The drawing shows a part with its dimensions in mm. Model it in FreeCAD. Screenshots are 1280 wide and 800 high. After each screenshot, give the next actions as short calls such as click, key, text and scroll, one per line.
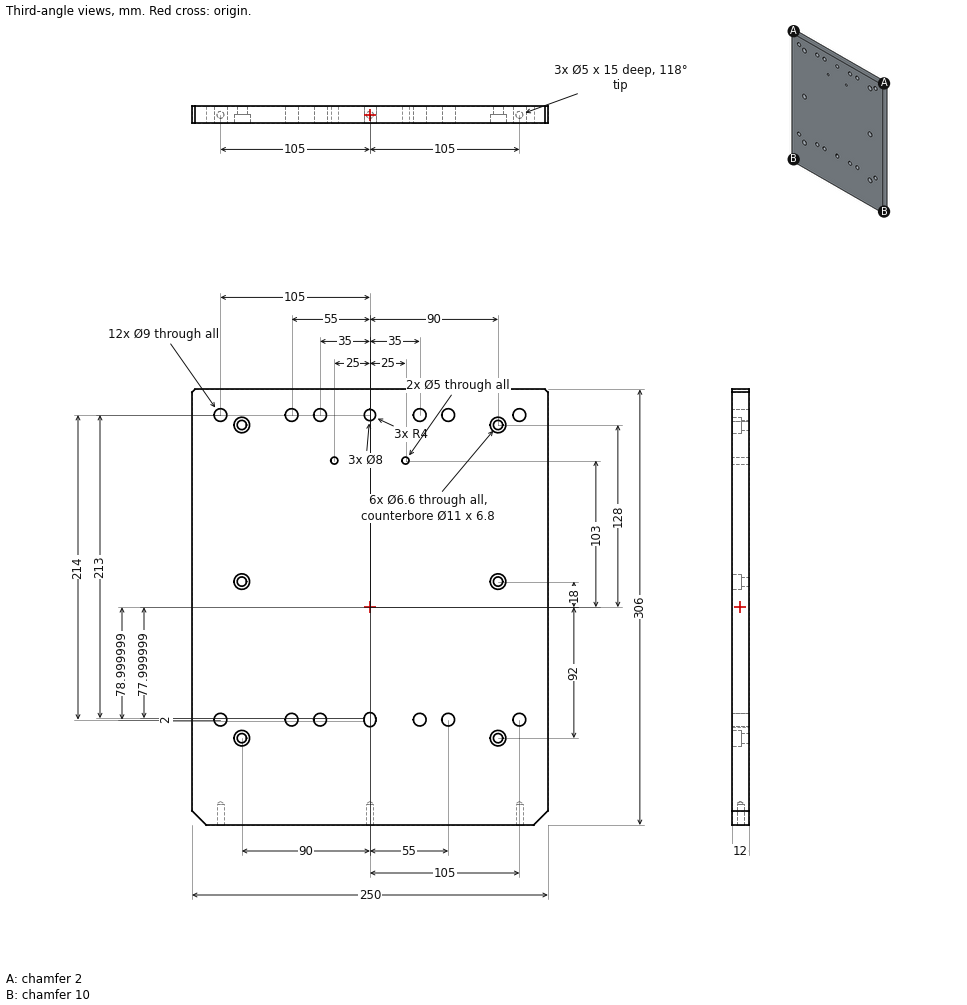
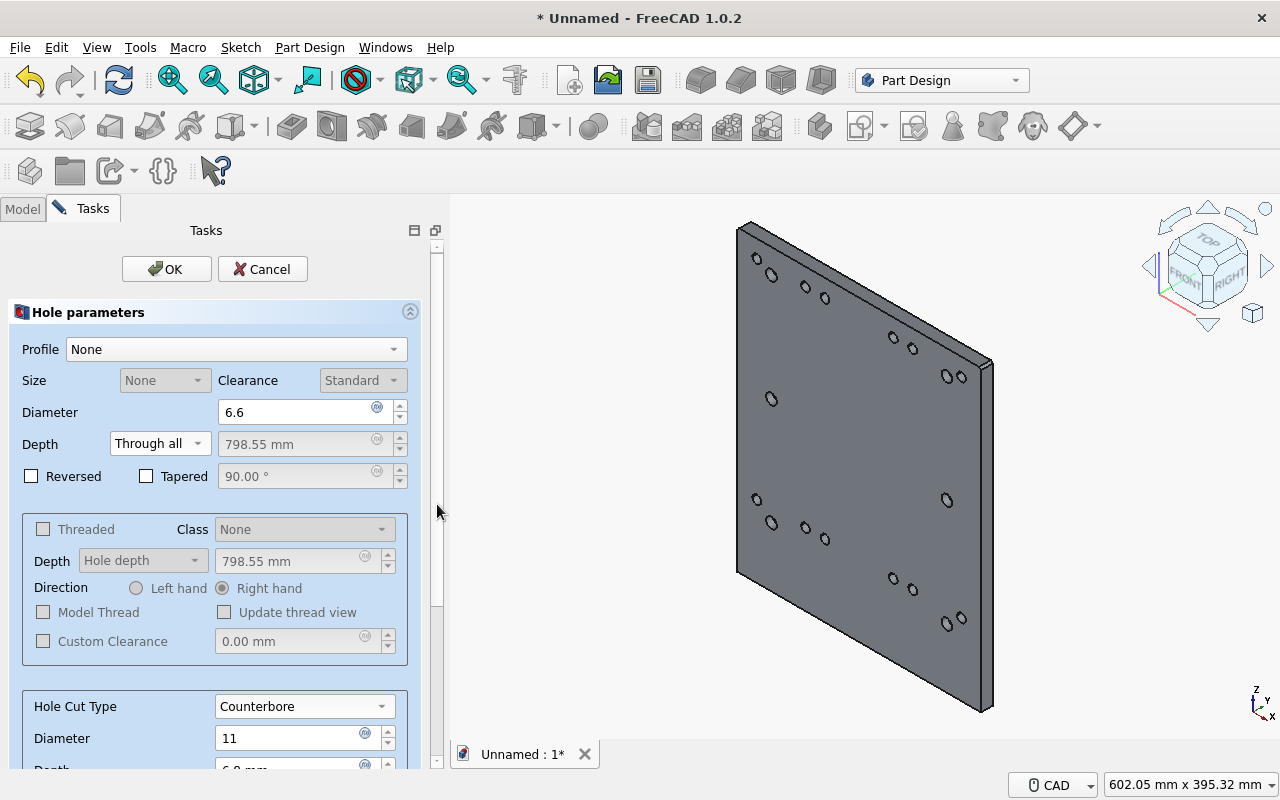
click(167, 269)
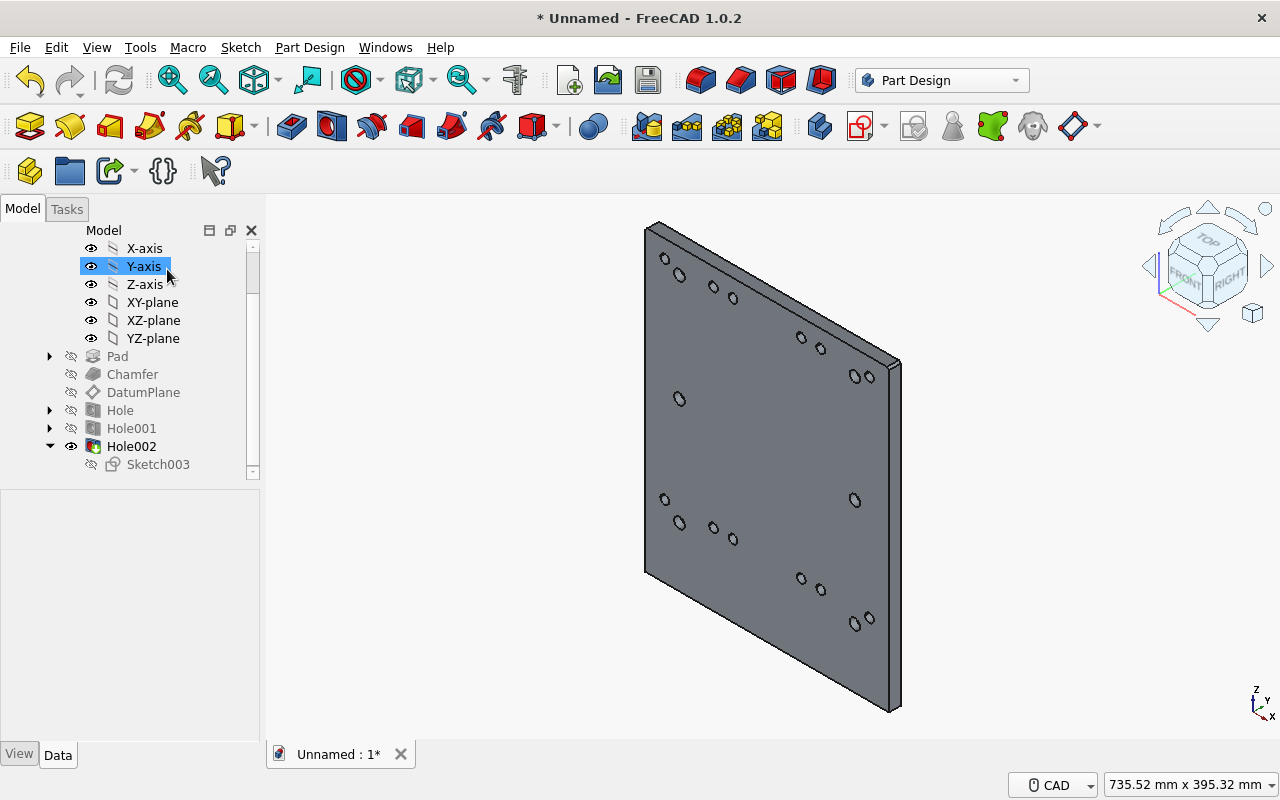
key(4)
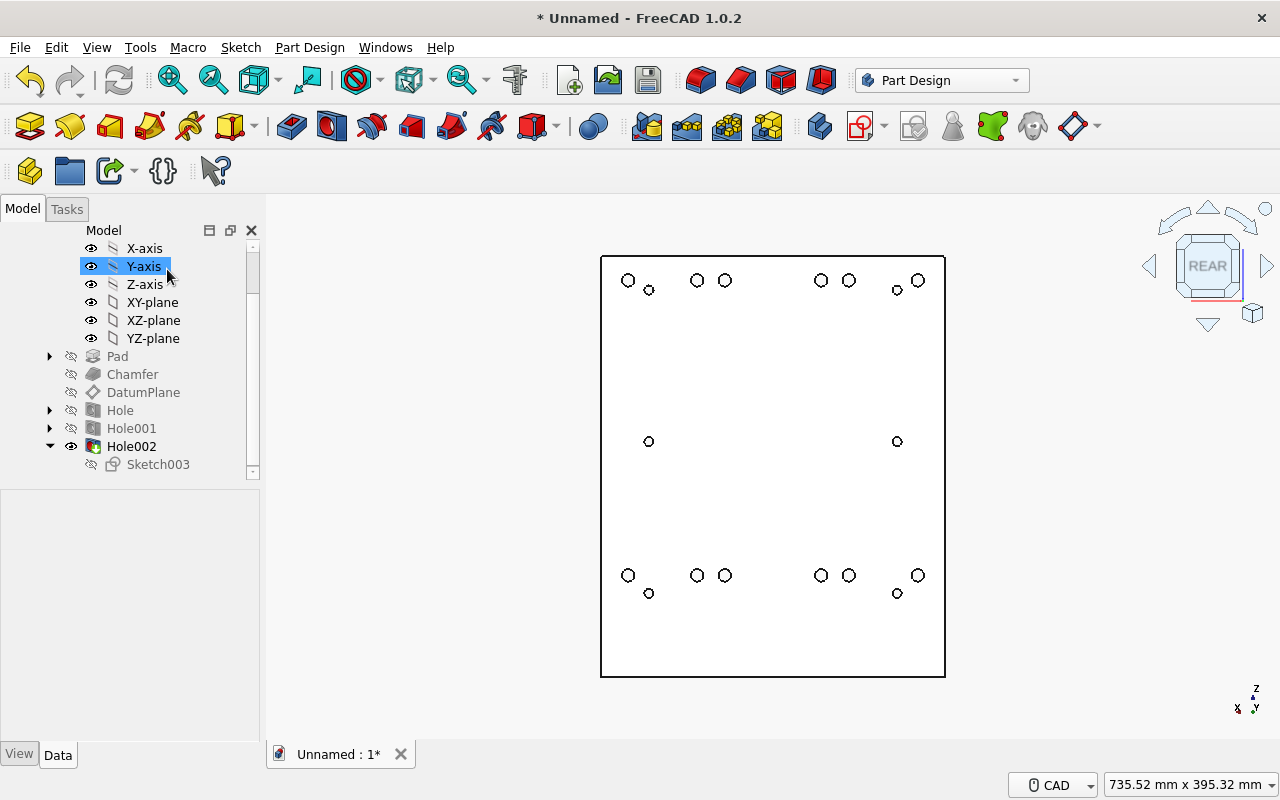
click(773, 405)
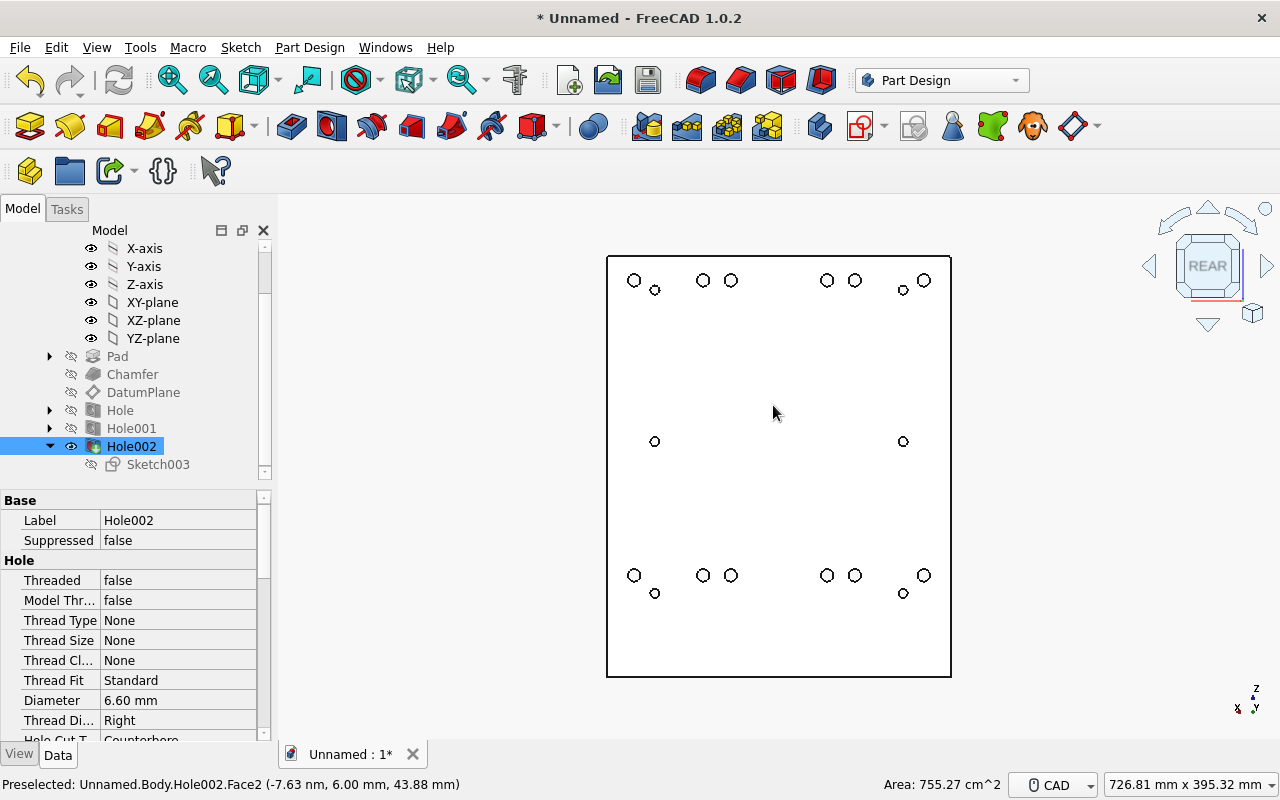
click(860, 126)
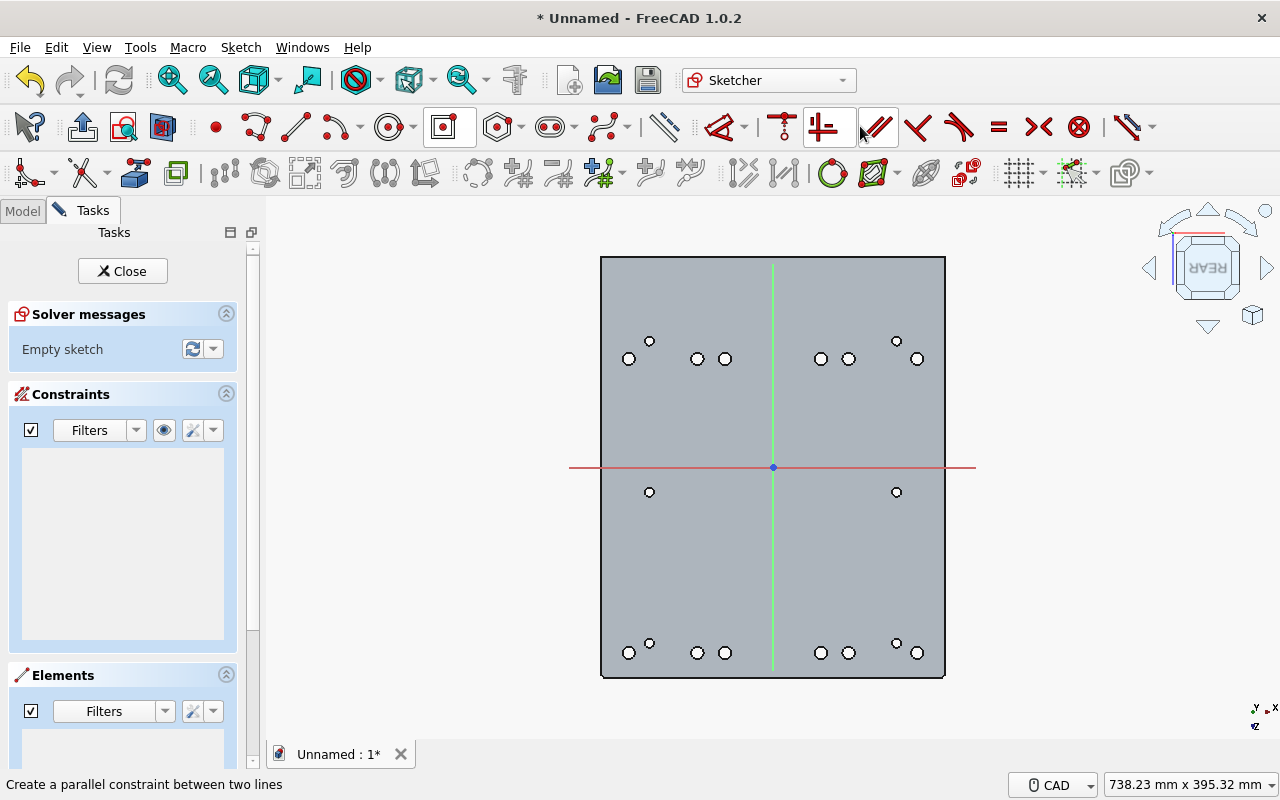
click(550, 128)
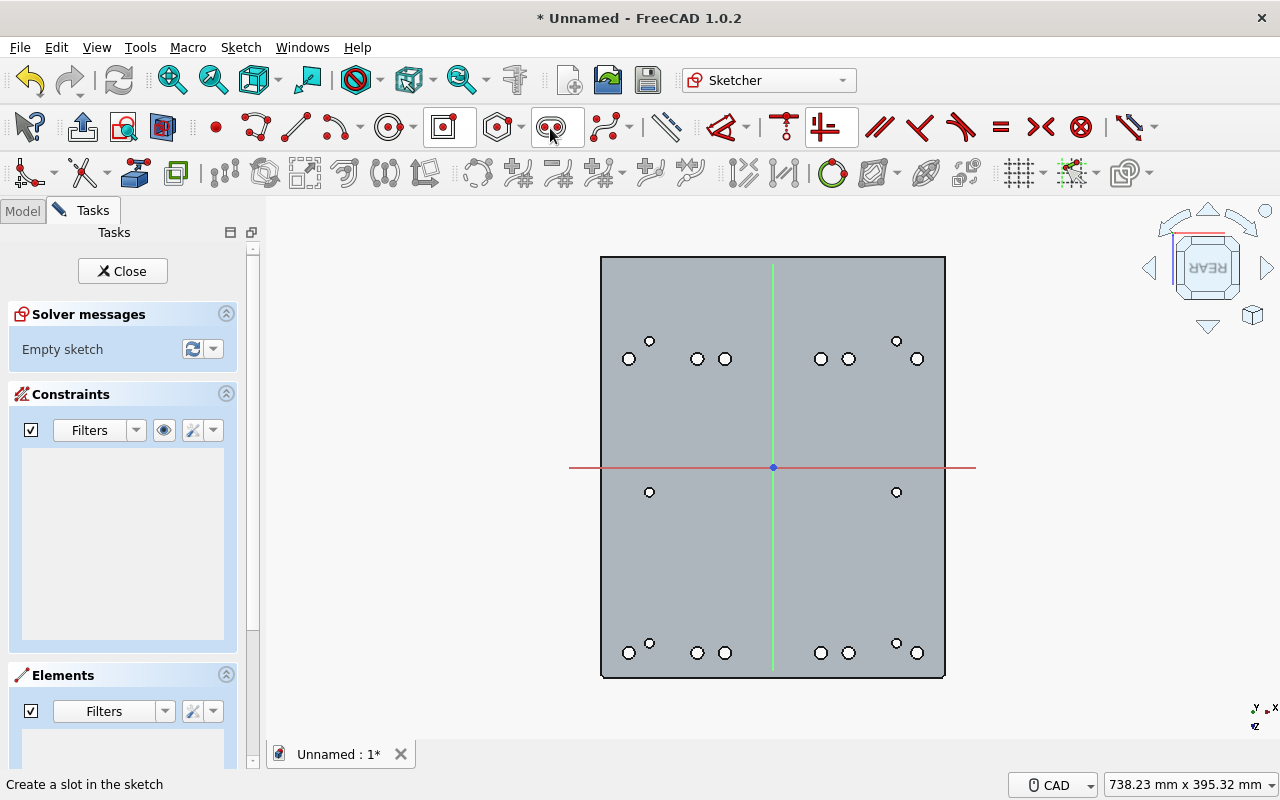
scroll(773, 360, up, 8)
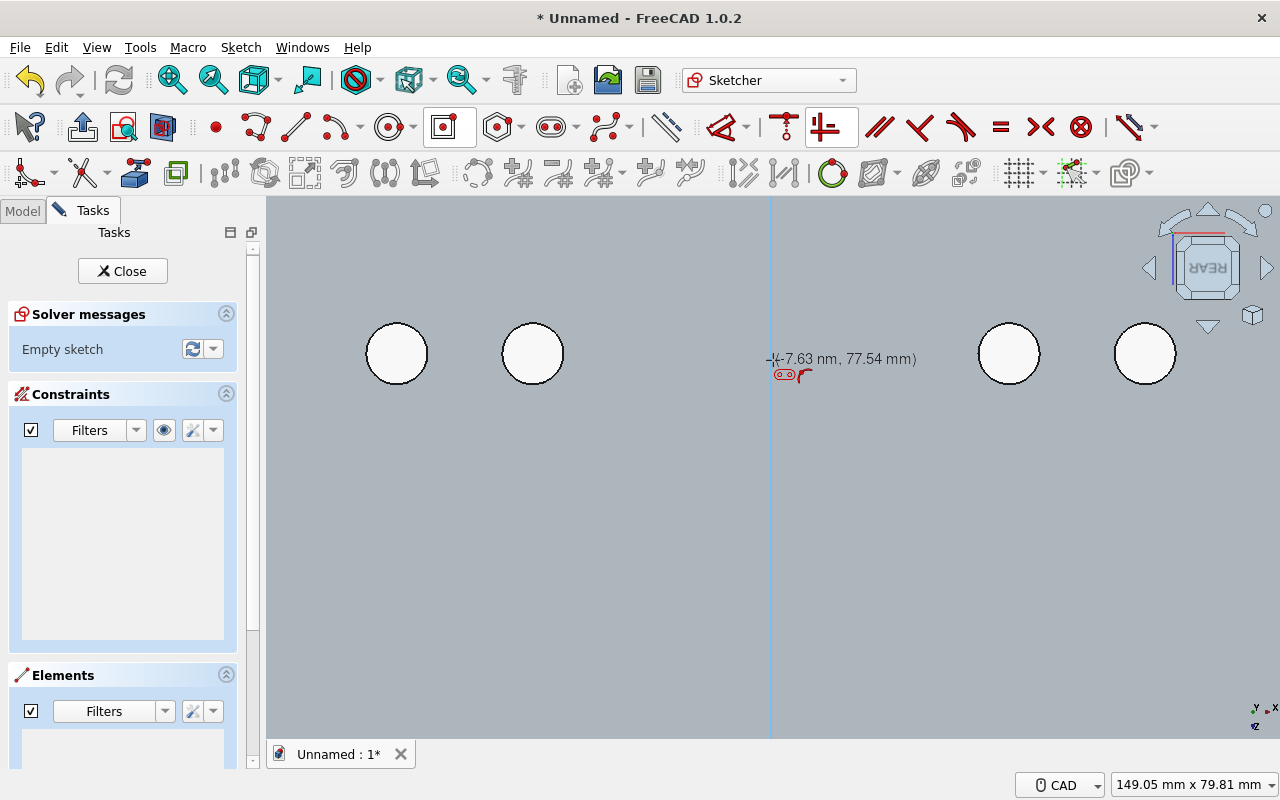
scroll(683, 268, down, 7)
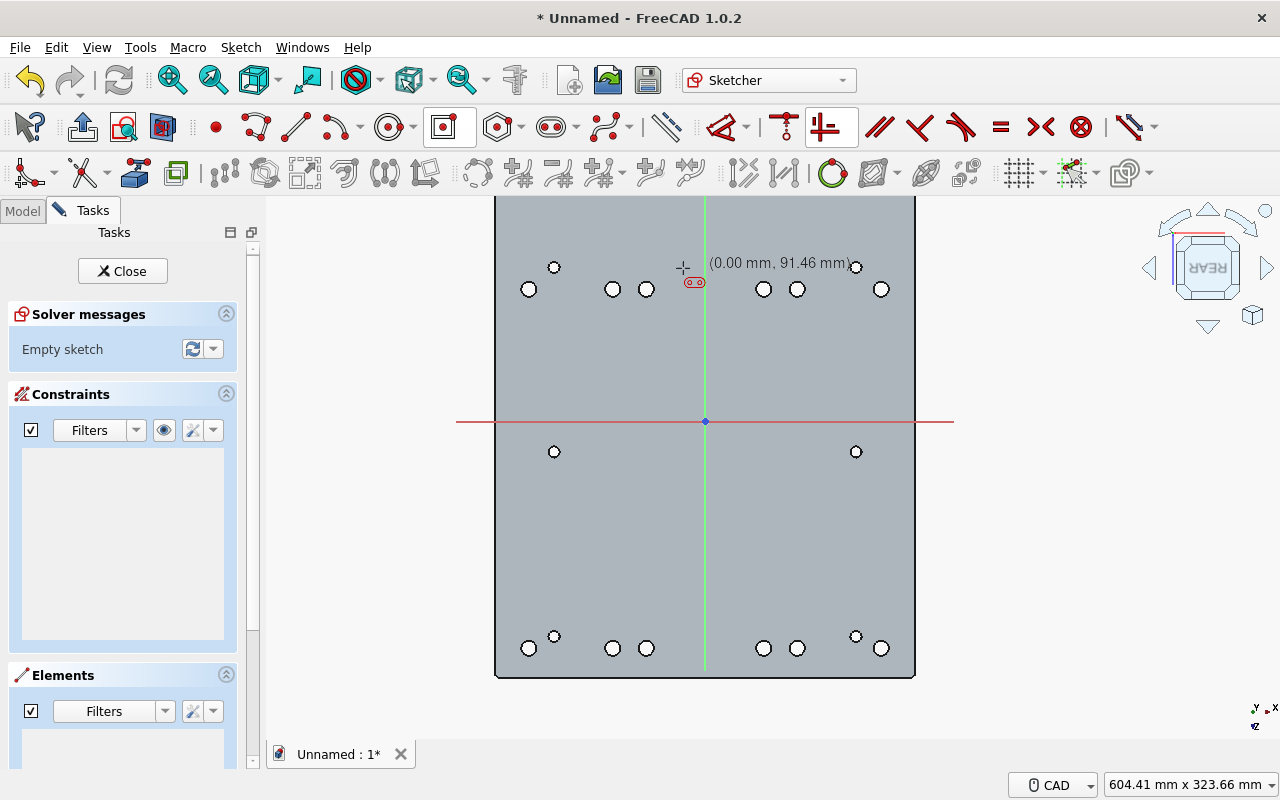
click(705, 291)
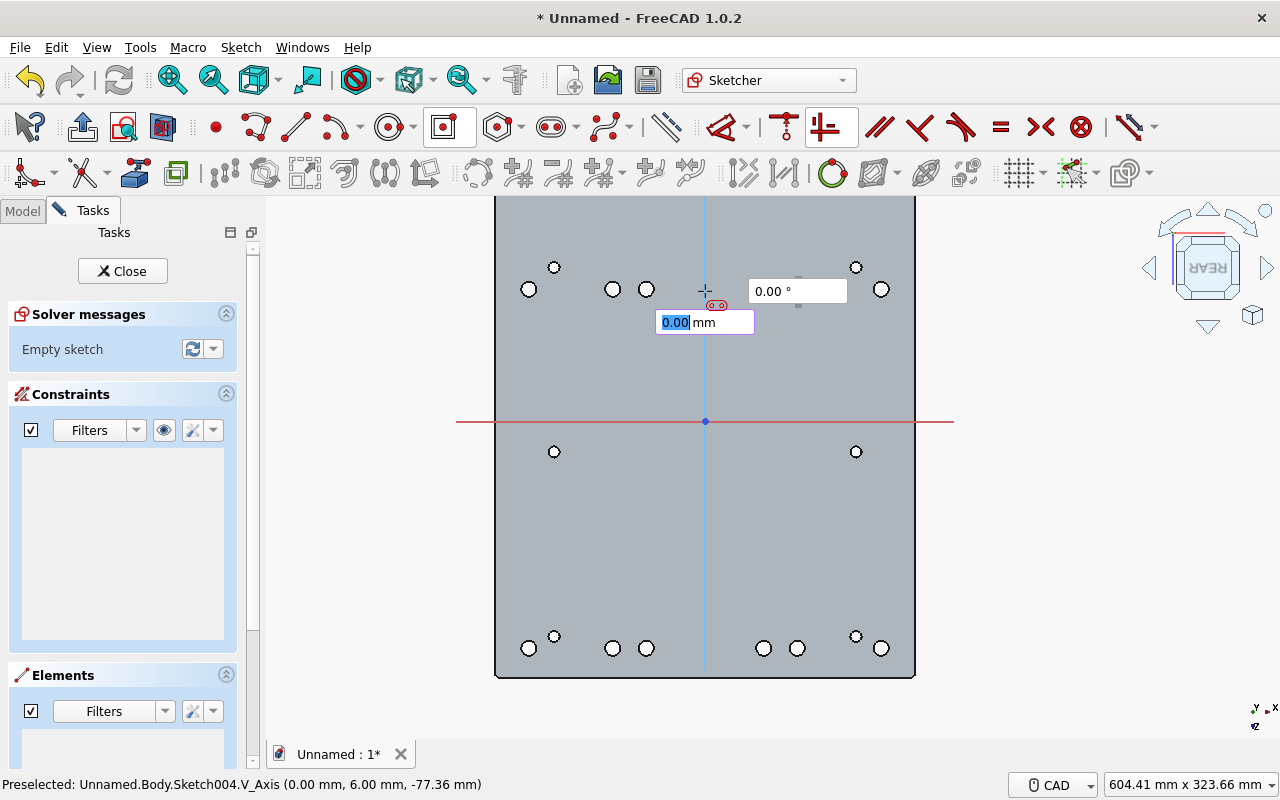
scroll(705, 288, up, 8)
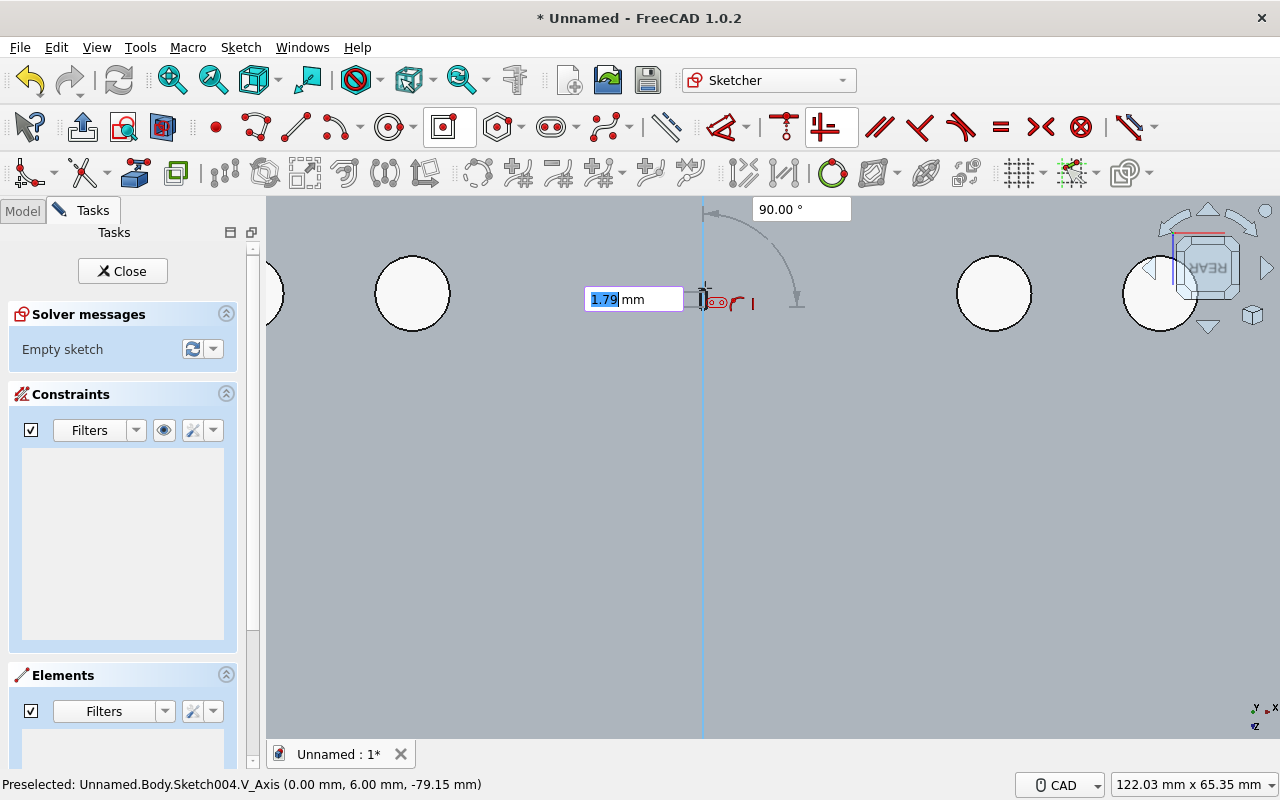
click(712, 285)